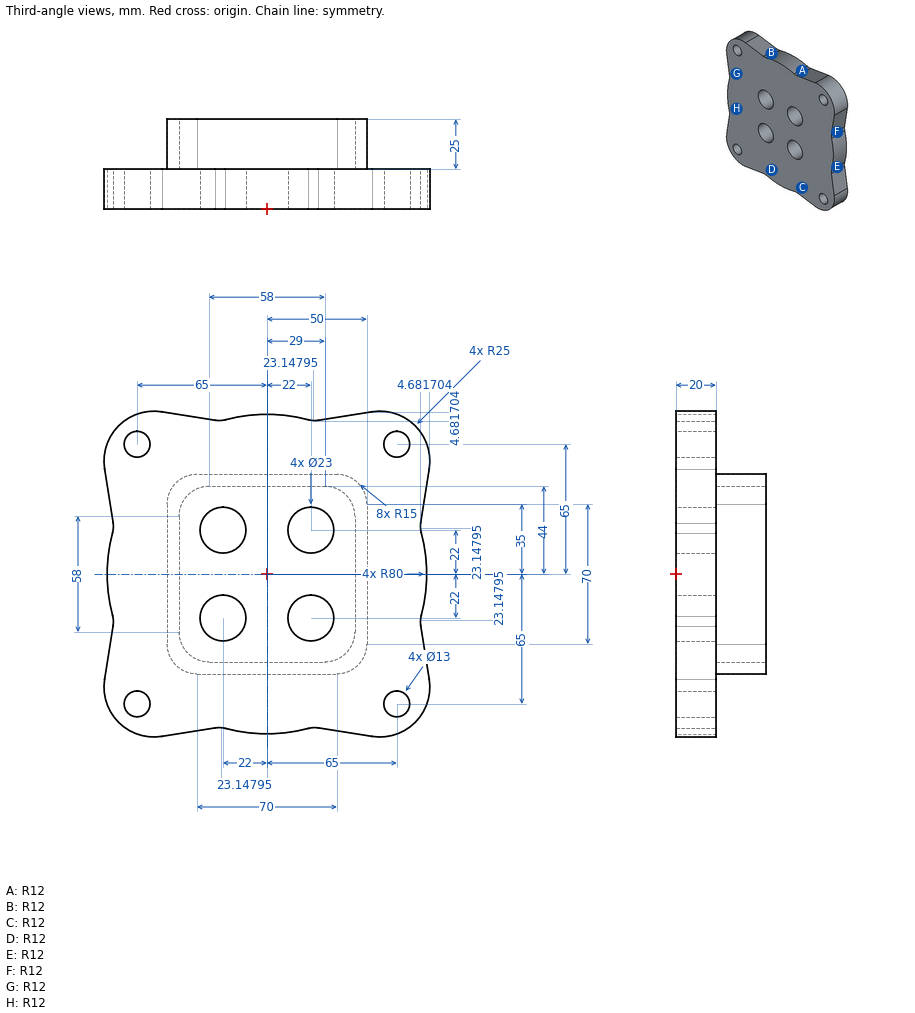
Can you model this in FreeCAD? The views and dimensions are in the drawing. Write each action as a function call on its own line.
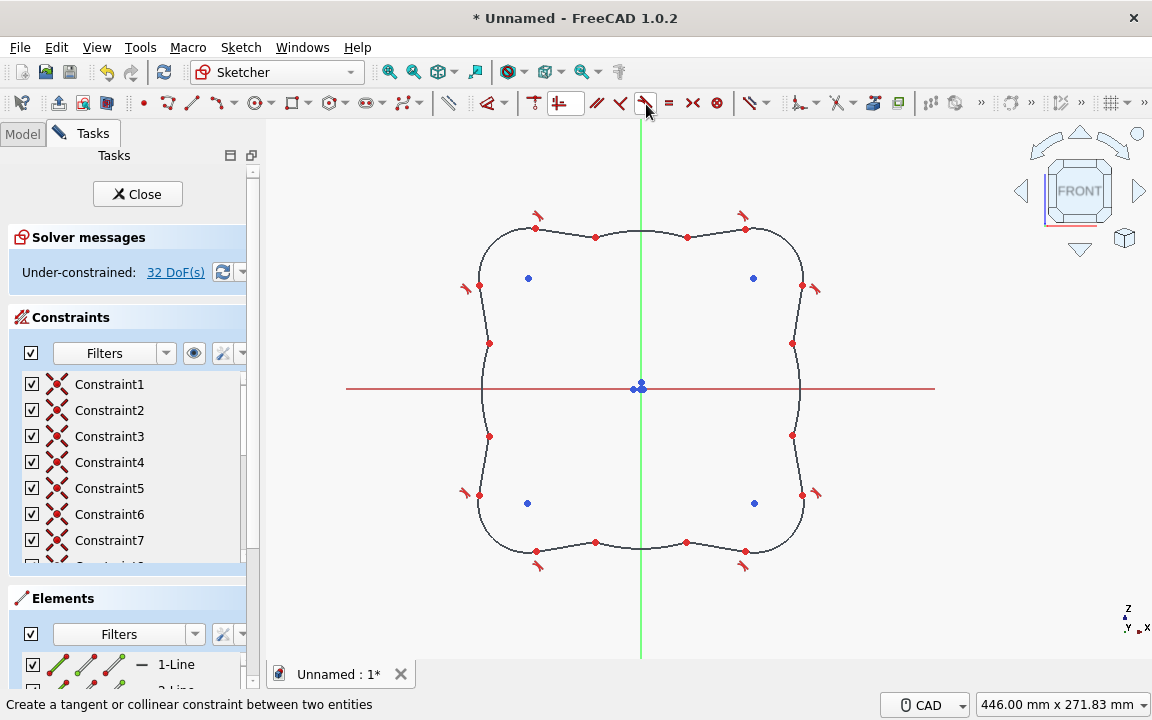
click(799, 409)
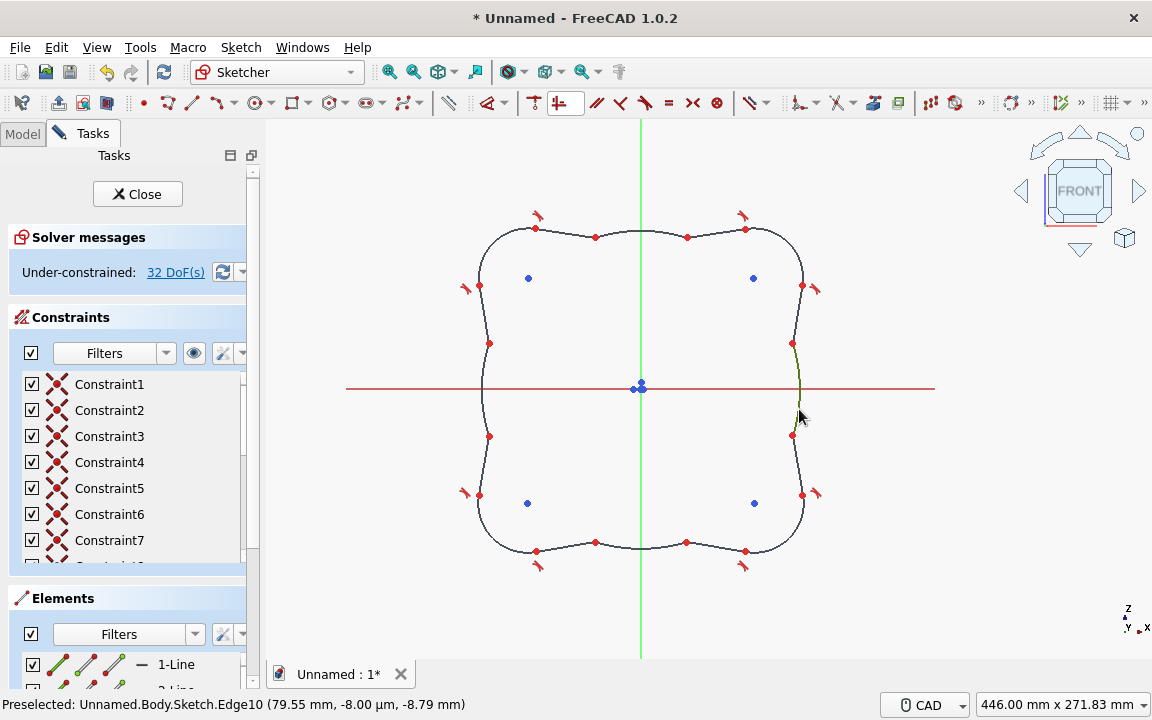
click(622, 548)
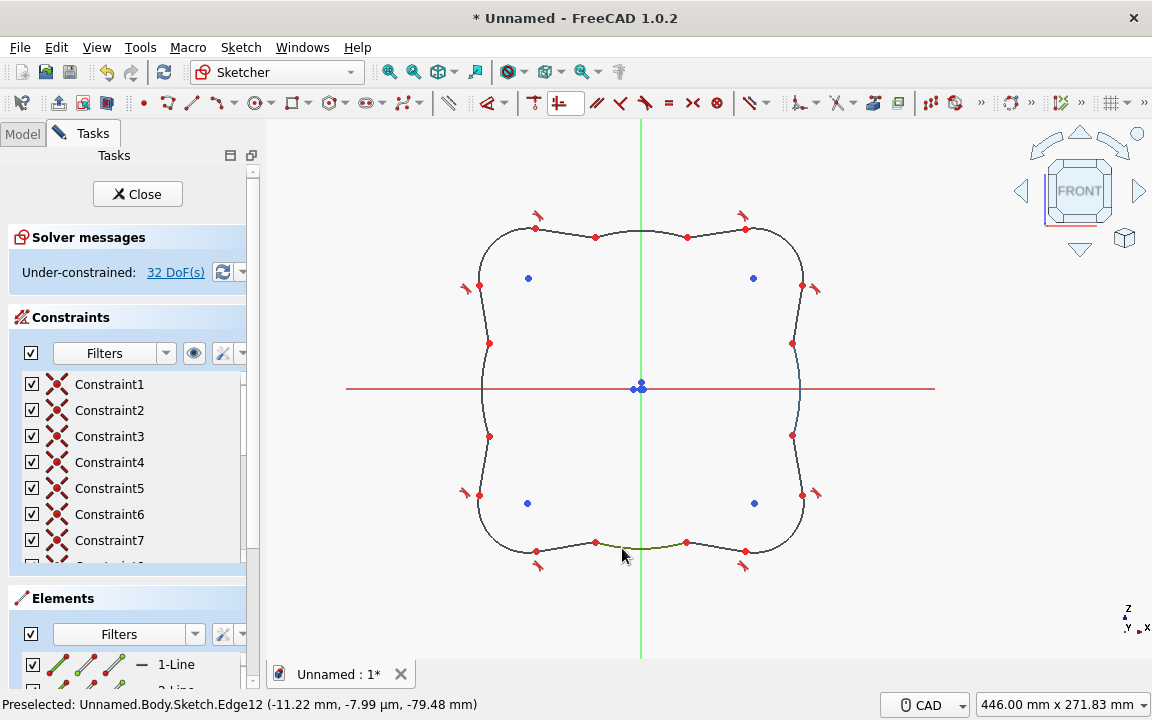
click(534, 104)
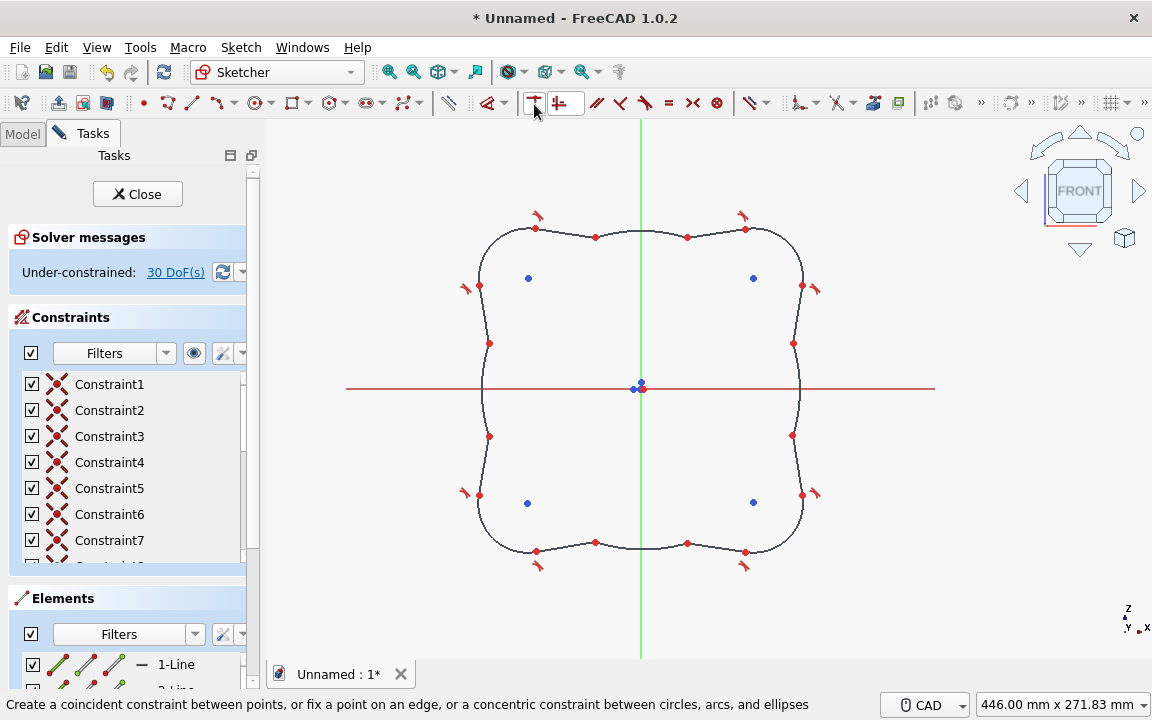
click(799, 409)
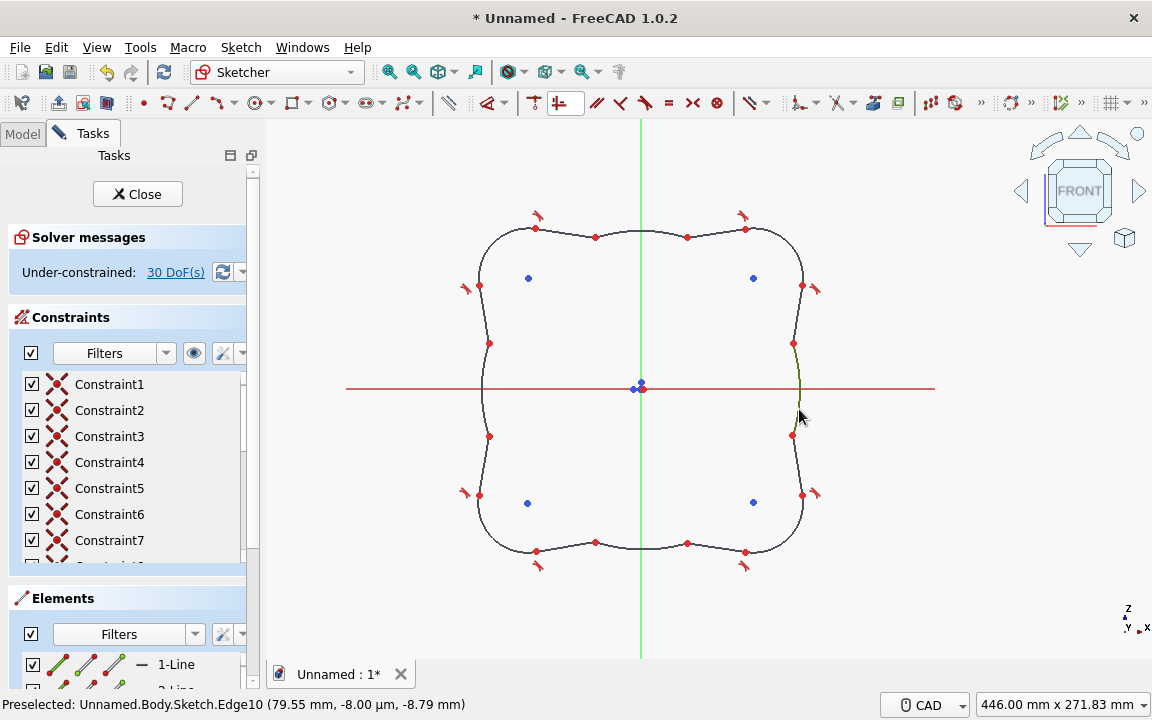
click(483, 371)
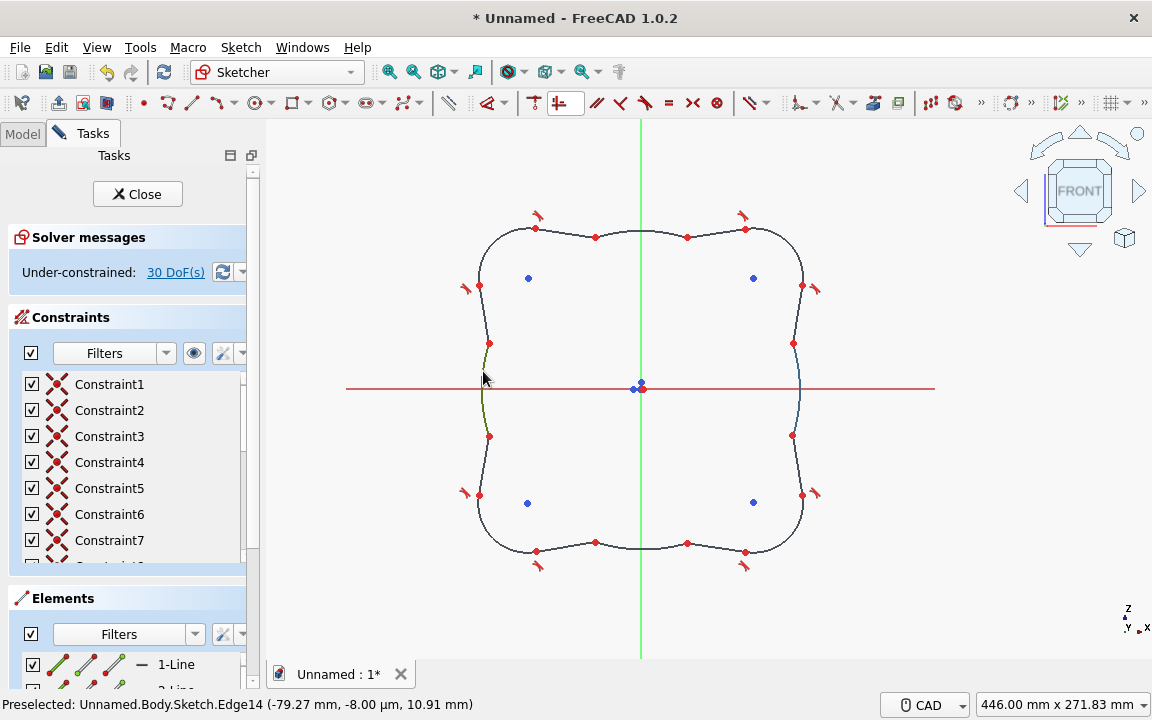
click(534, 104)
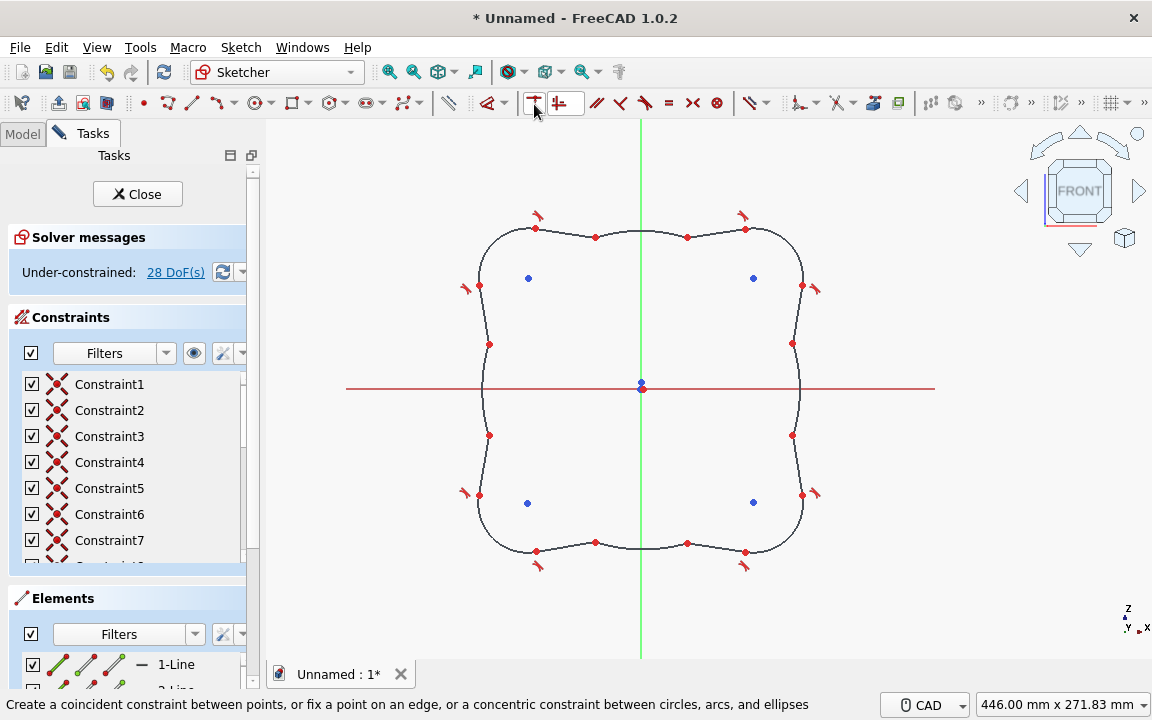
click(799, 409)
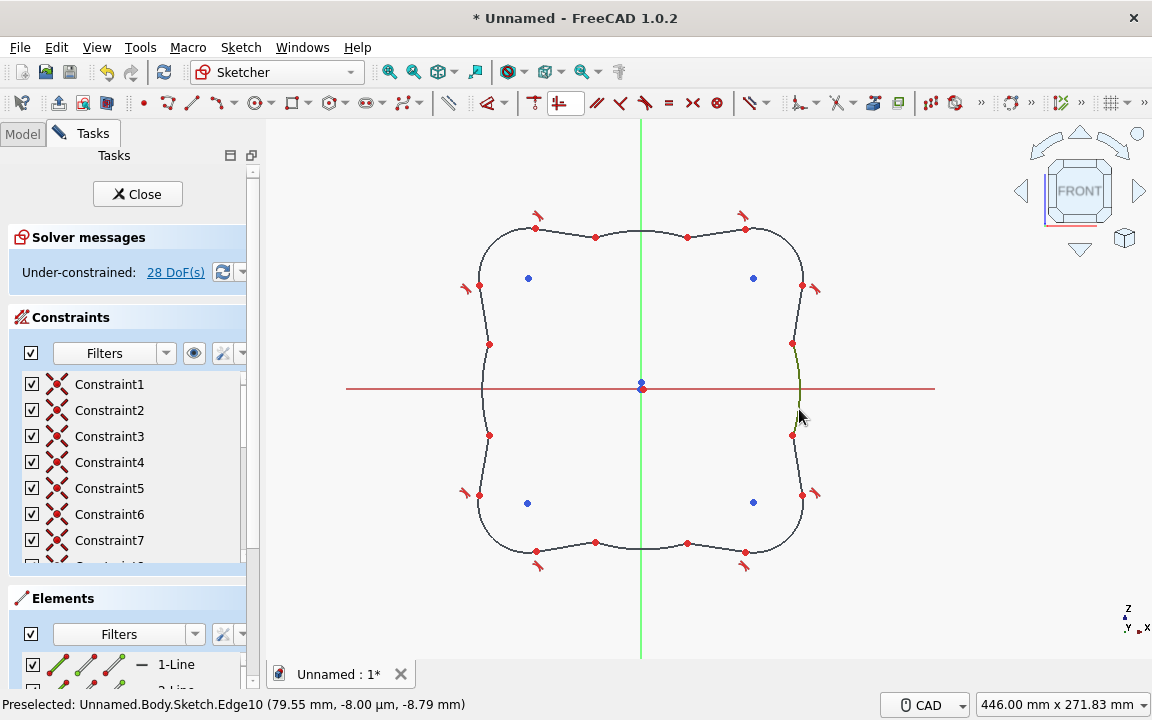
click(660, 232)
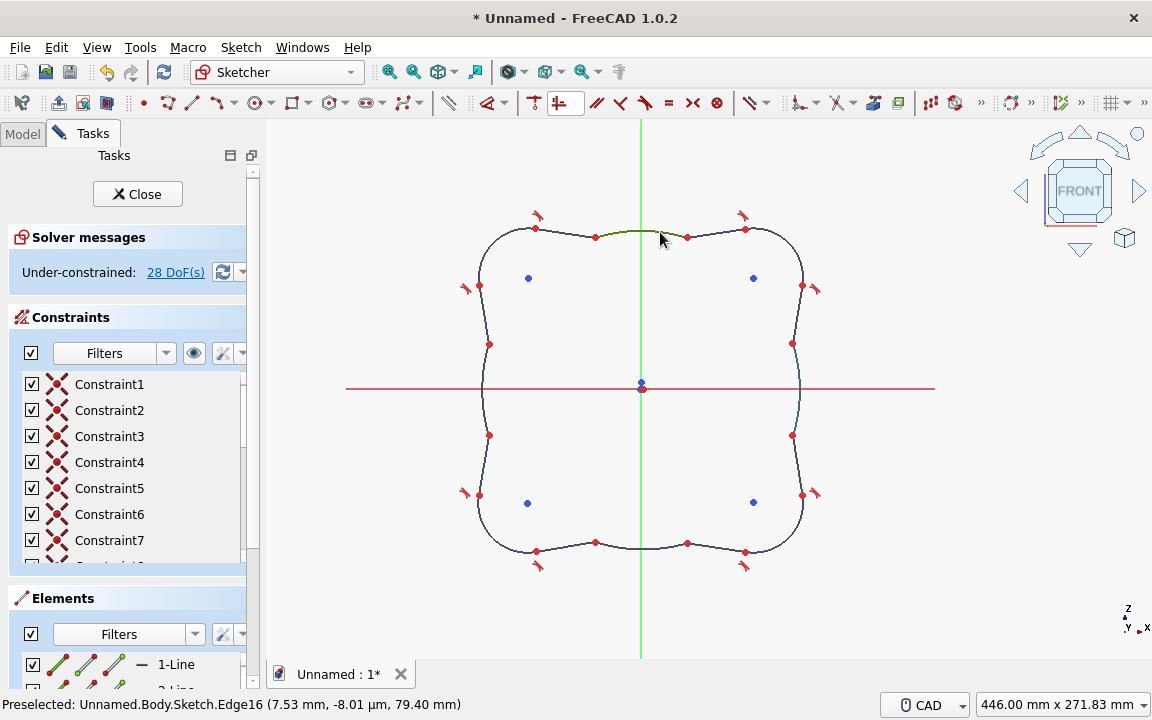
click(534, 104)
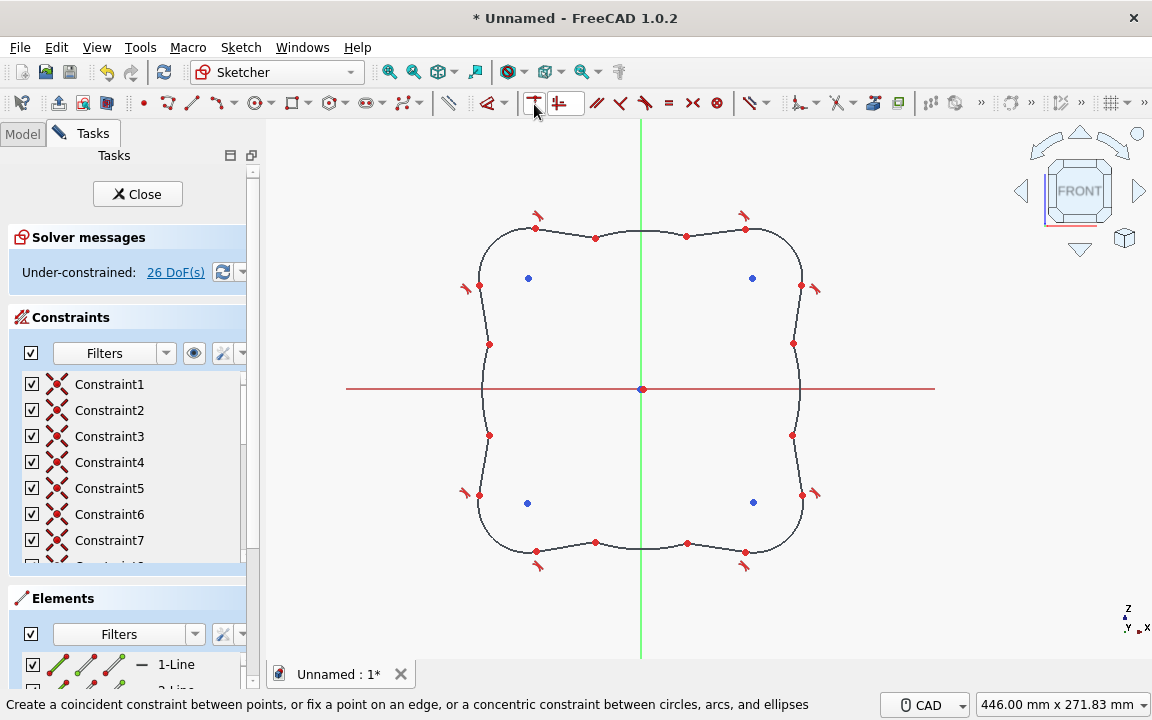
drag(631, 379, 653, 400)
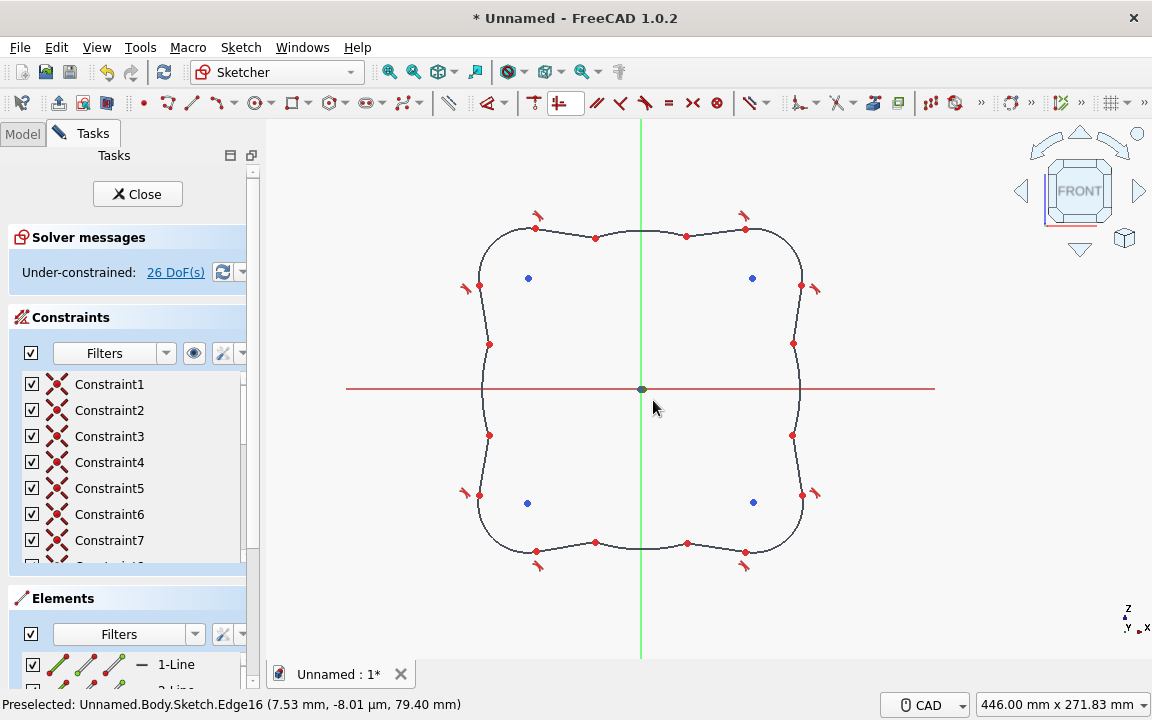
click(534, 104)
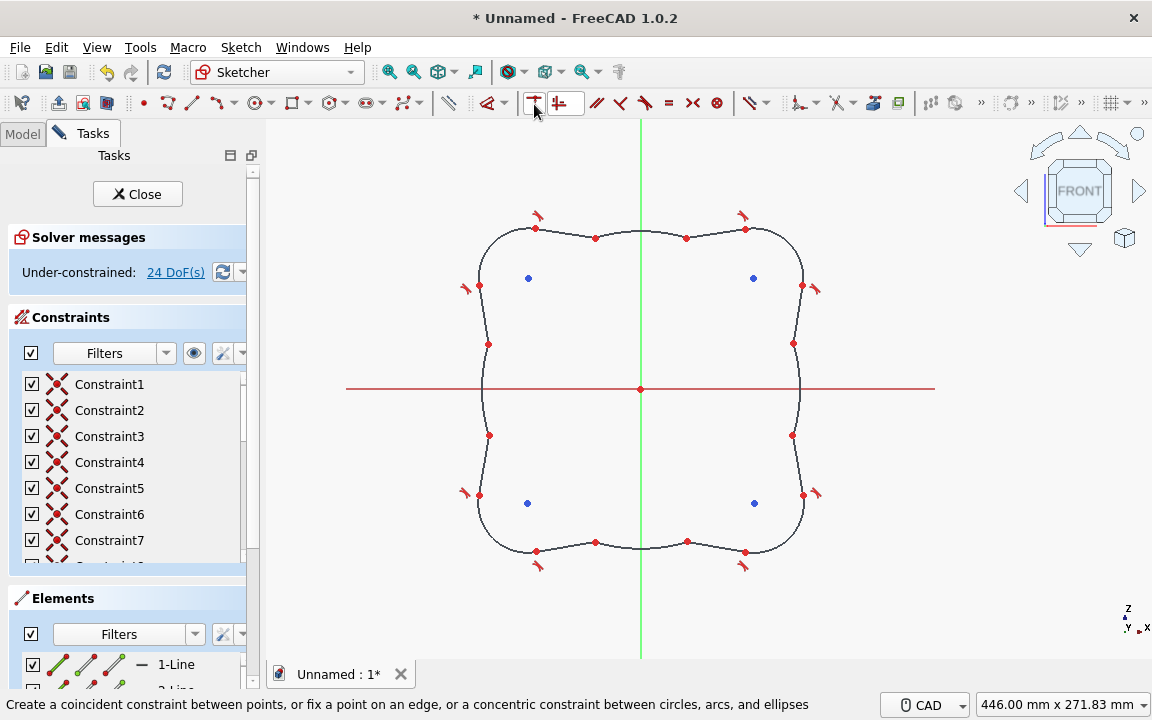
click(799, 259)